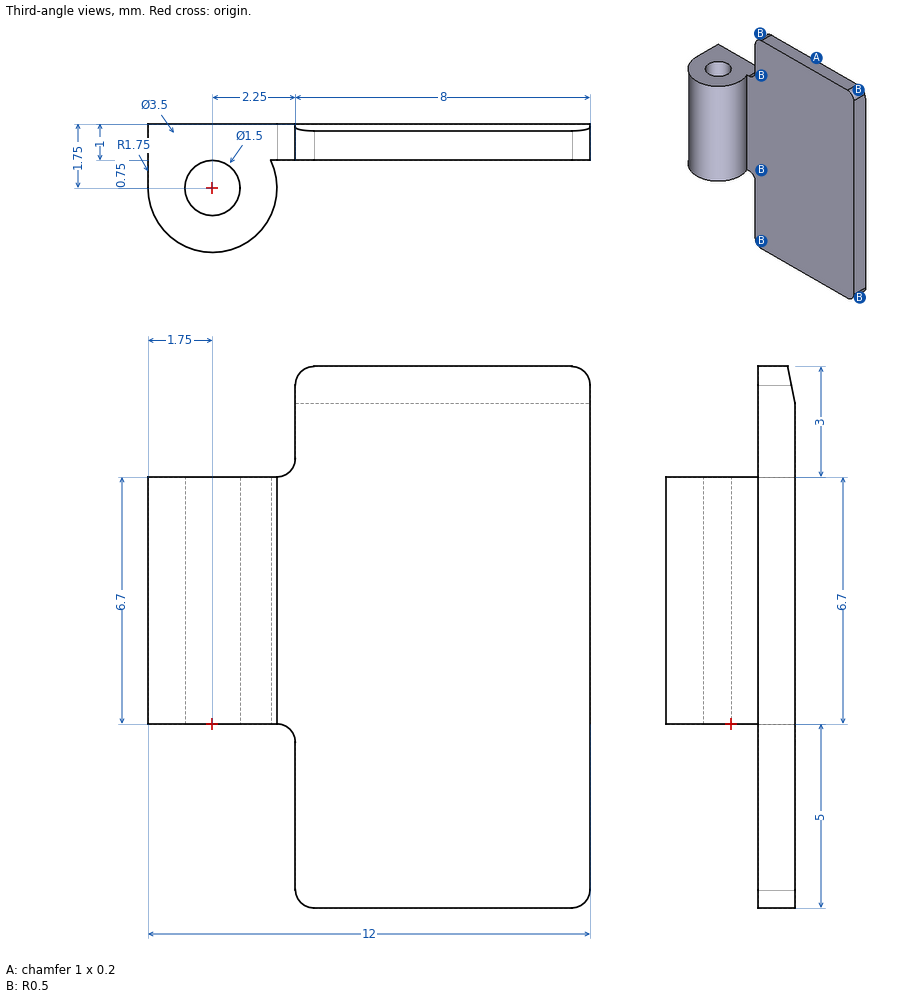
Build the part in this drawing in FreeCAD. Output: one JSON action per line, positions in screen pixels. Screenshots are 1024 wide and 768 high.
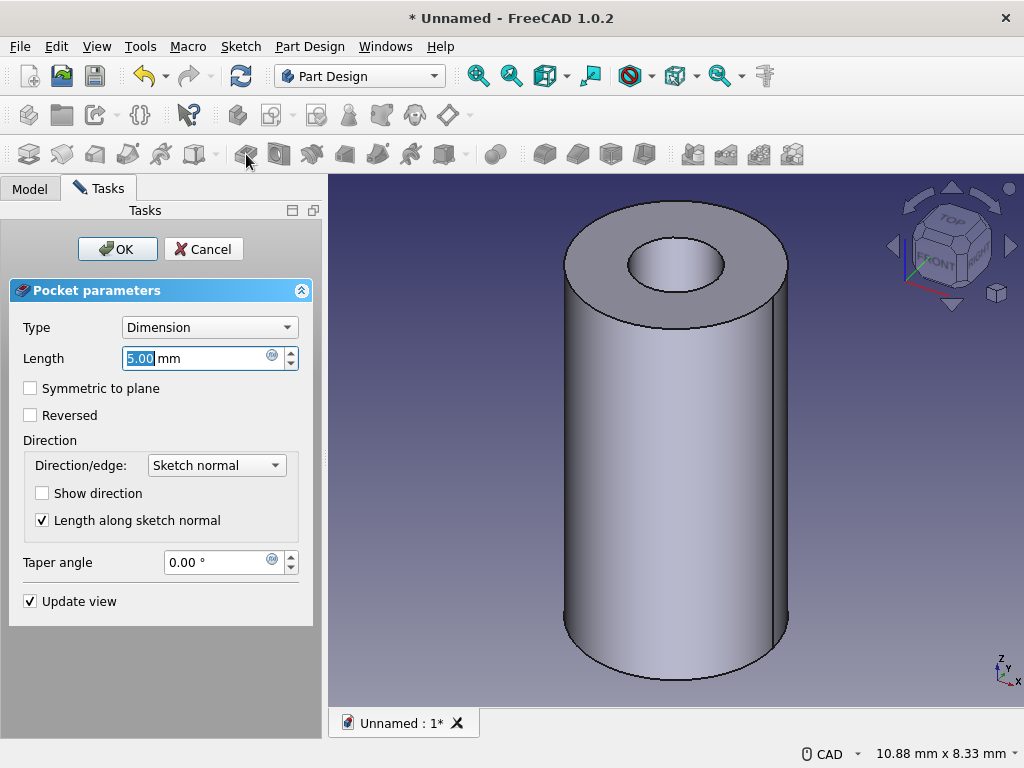
{"action": "left_click", "coordinate": [210, 328]}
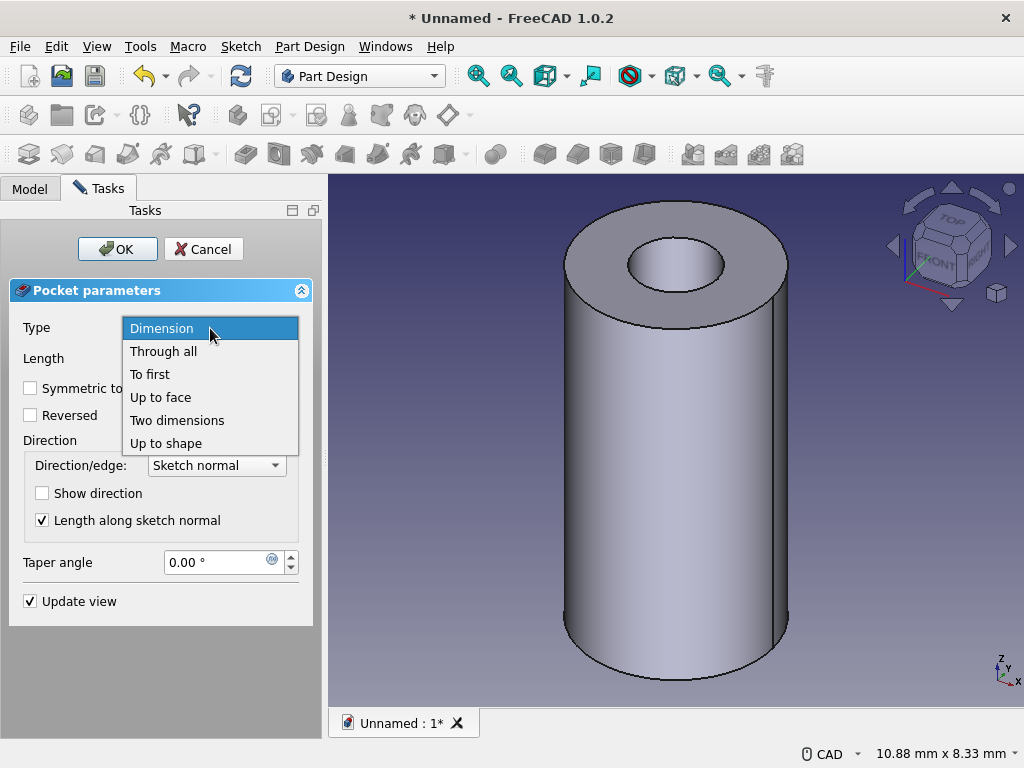
{"action": "left_click", "coordinate": [208, 352]}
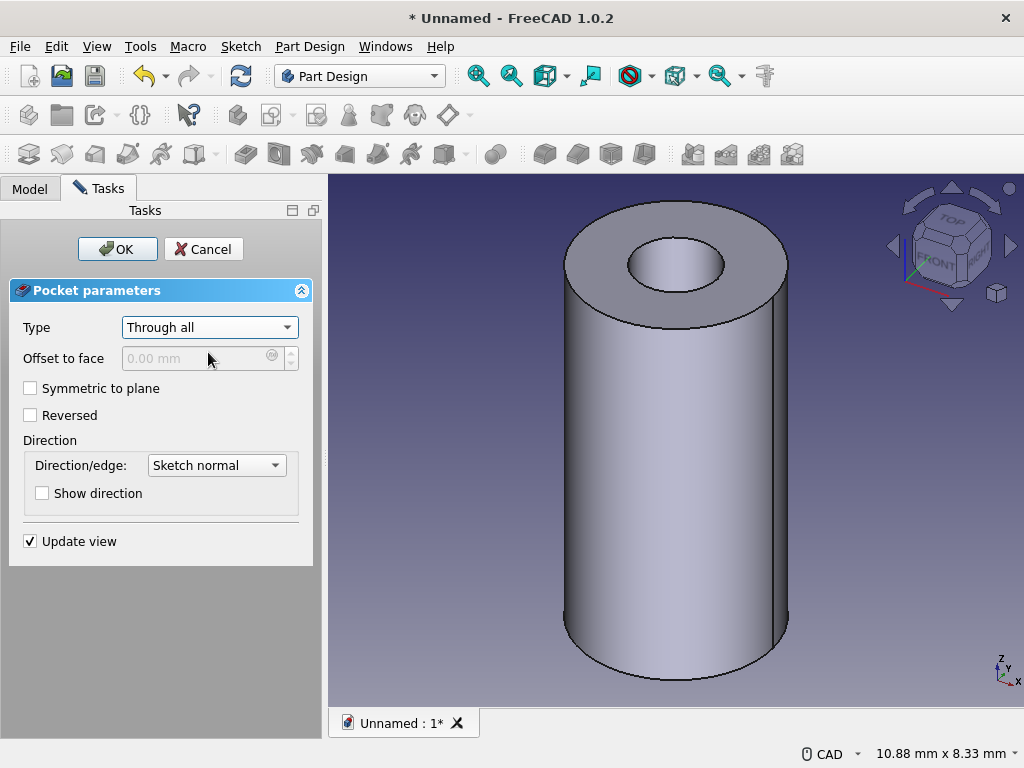
{"action": "left_click", "coordinate": [118, 249]}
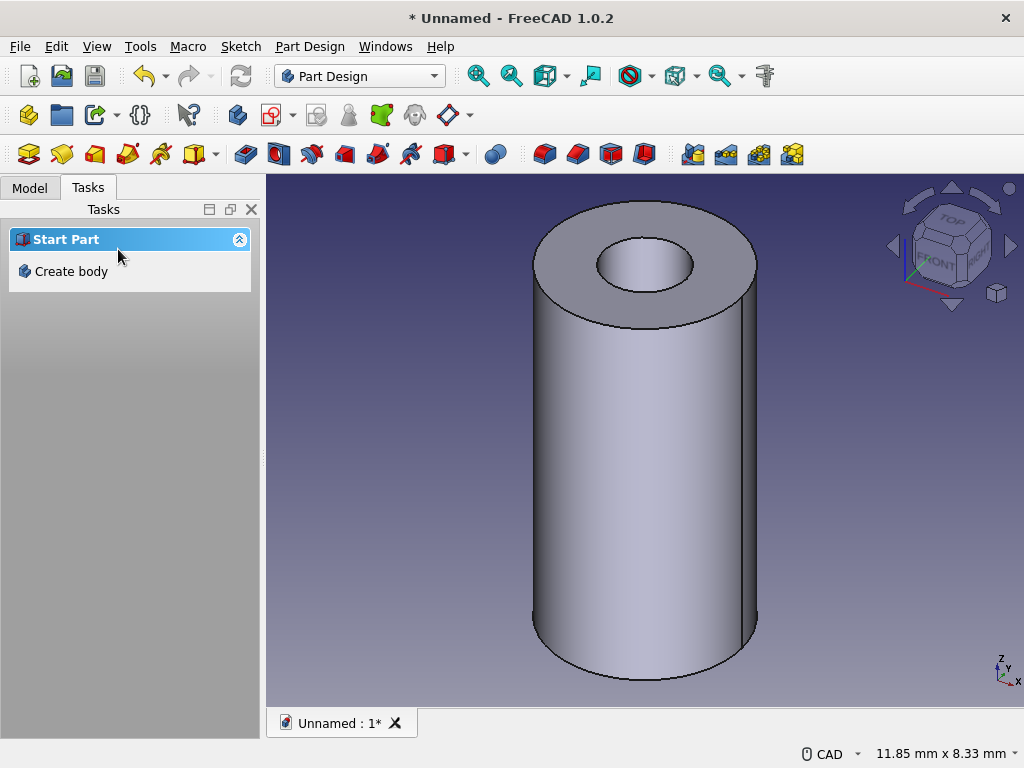
{"action": "left_click", "coordinate": [30, 188]}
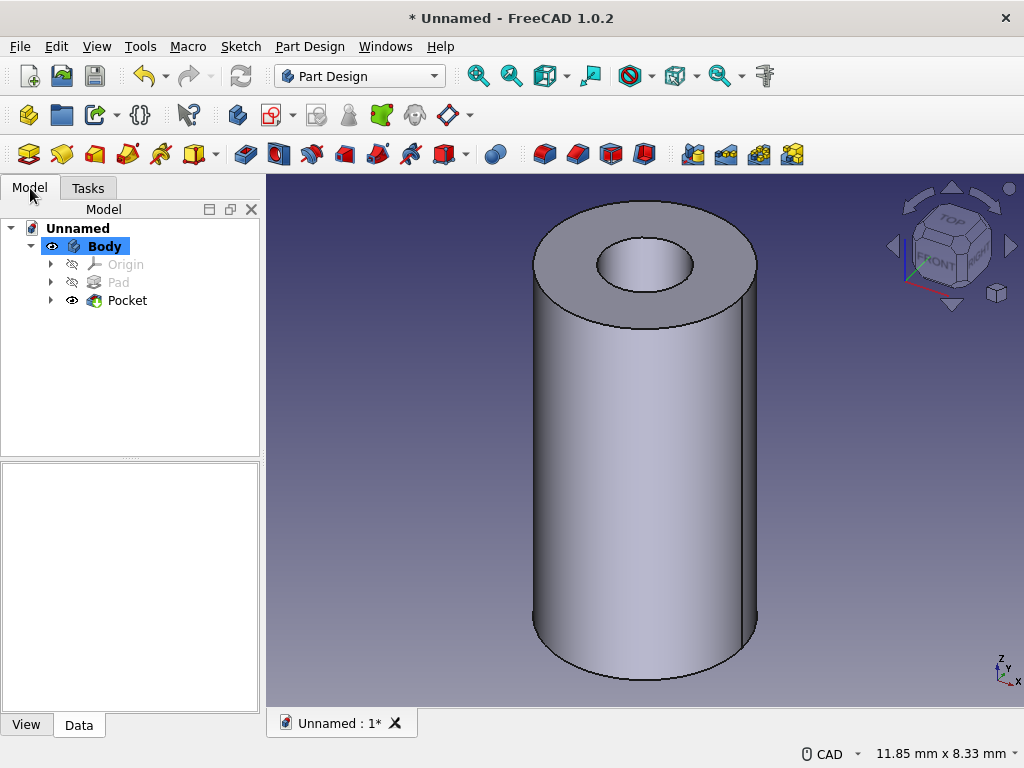
{"action": "left_click", "coordinate": [51, 264]}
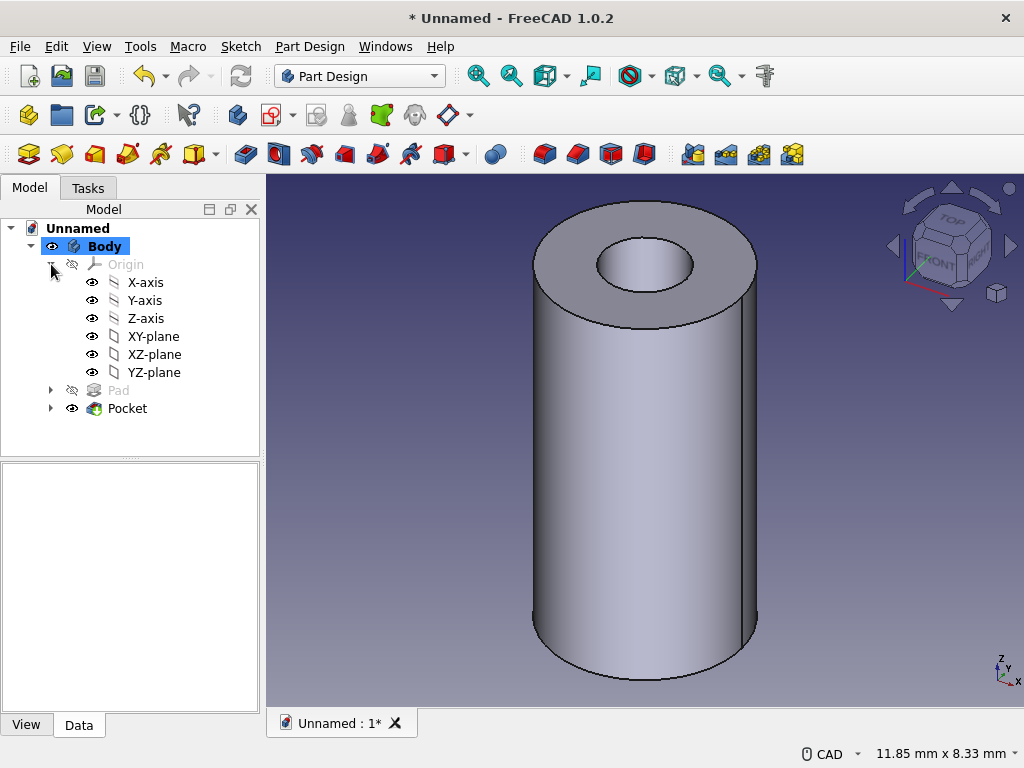
{"action": "left_click", "coordinate": [137, 354]}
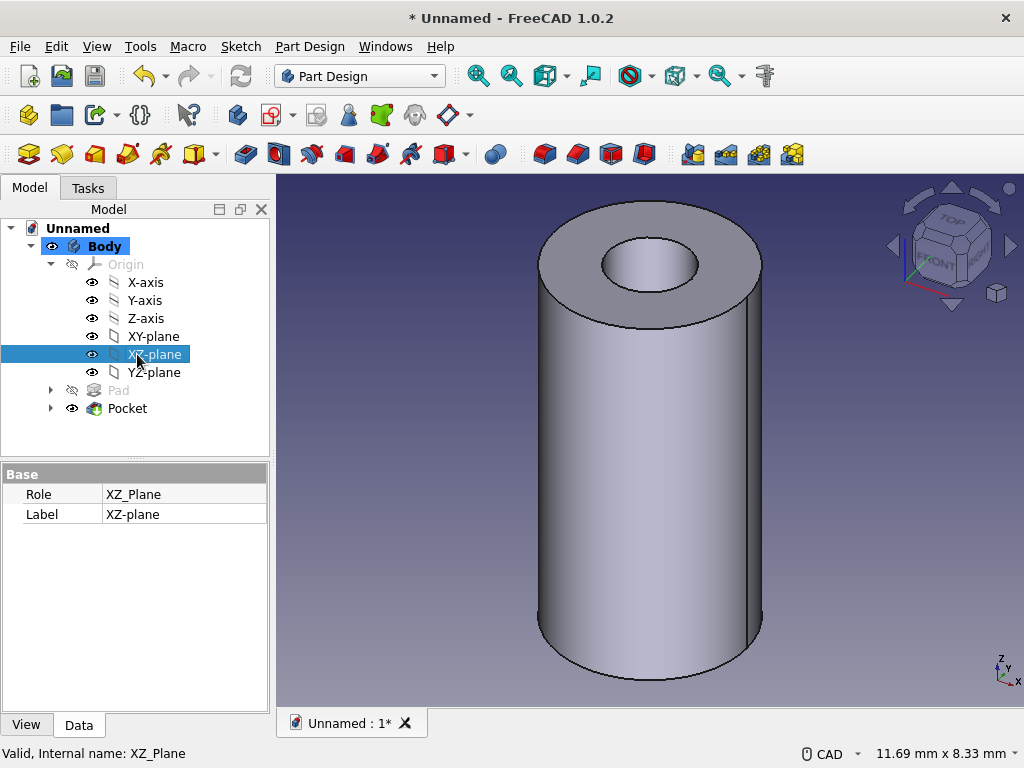
{"action": "left_click", "coordinate": [448, 116]}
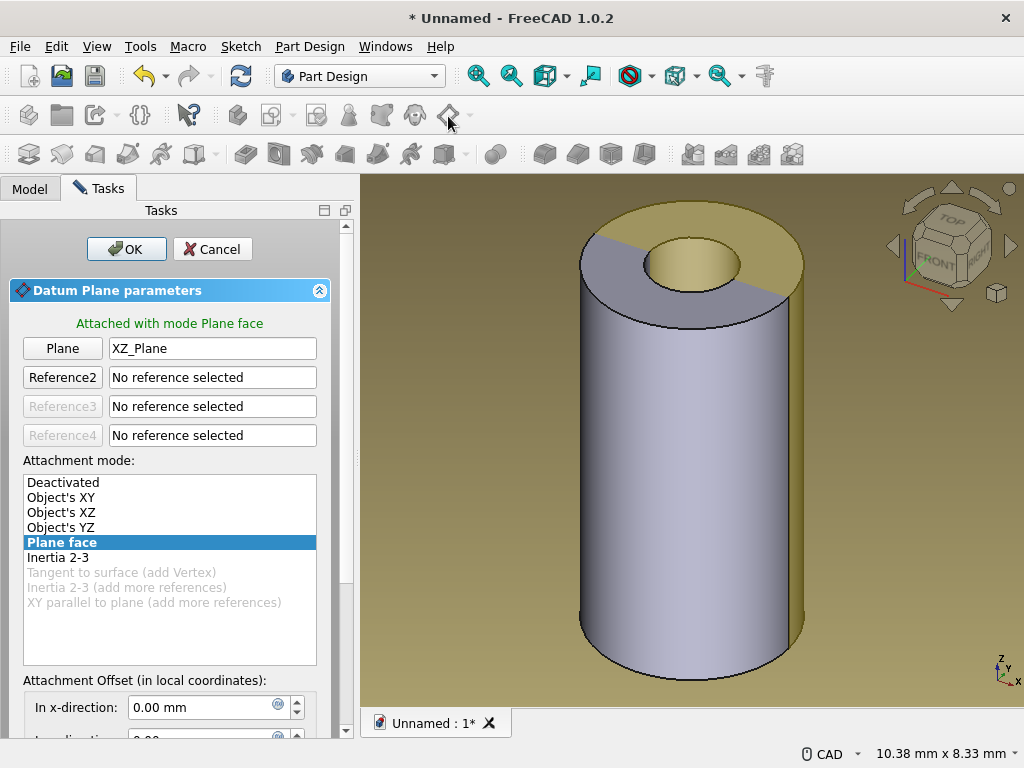
{"action": "scroll", "coordinate": [346, 479], "scroll_direction": "down", "scroll_amount": 2}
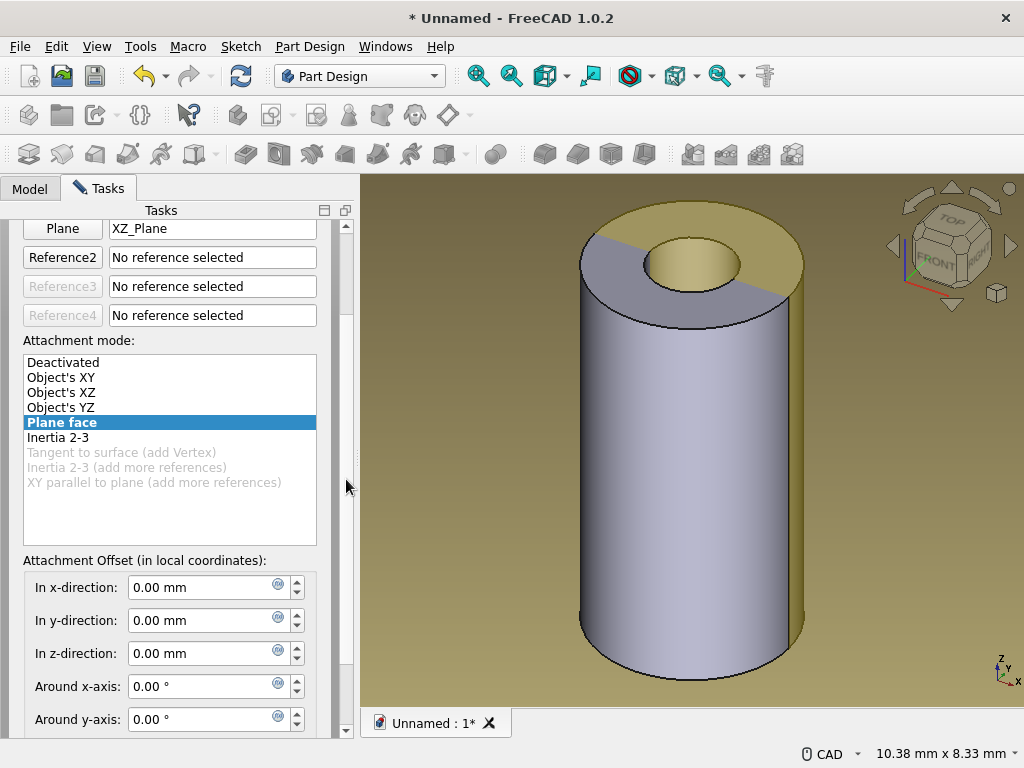
{"action": "triple_click", "coordinate": [210, 654]}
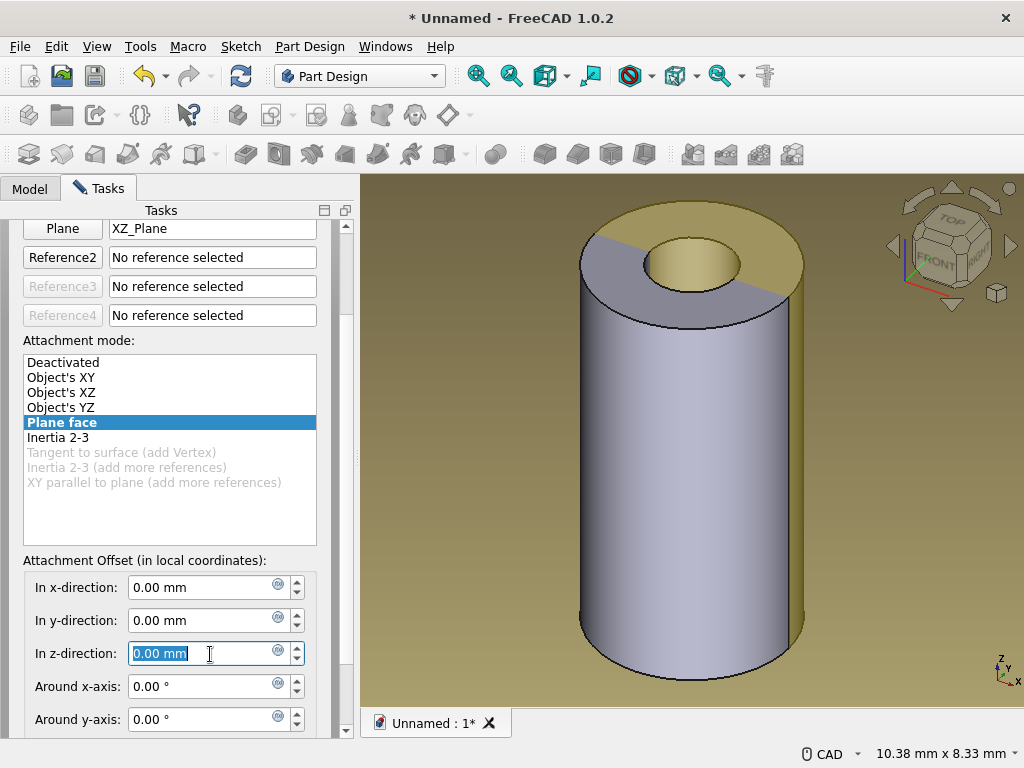
{"action": "type", "text": "-1.75"}
{"action": "key", "text": "Tab"}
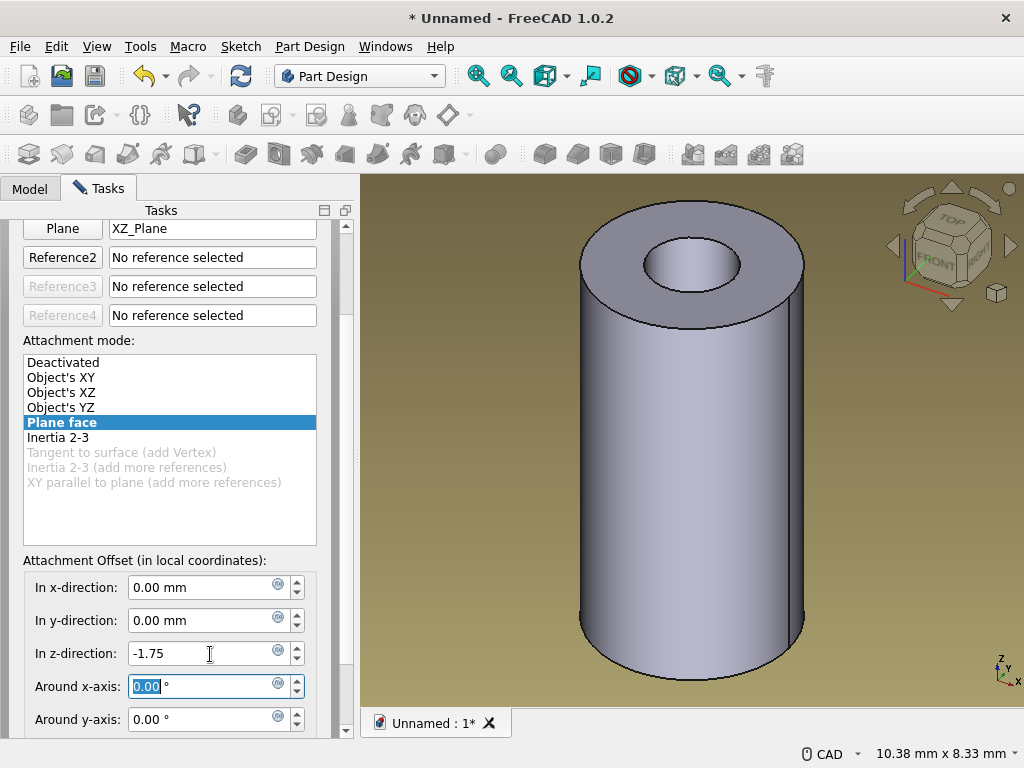
{"action": "scroll", "coordinate": [346, 479], "scroll_direction": "up", "scroll_amount": 3}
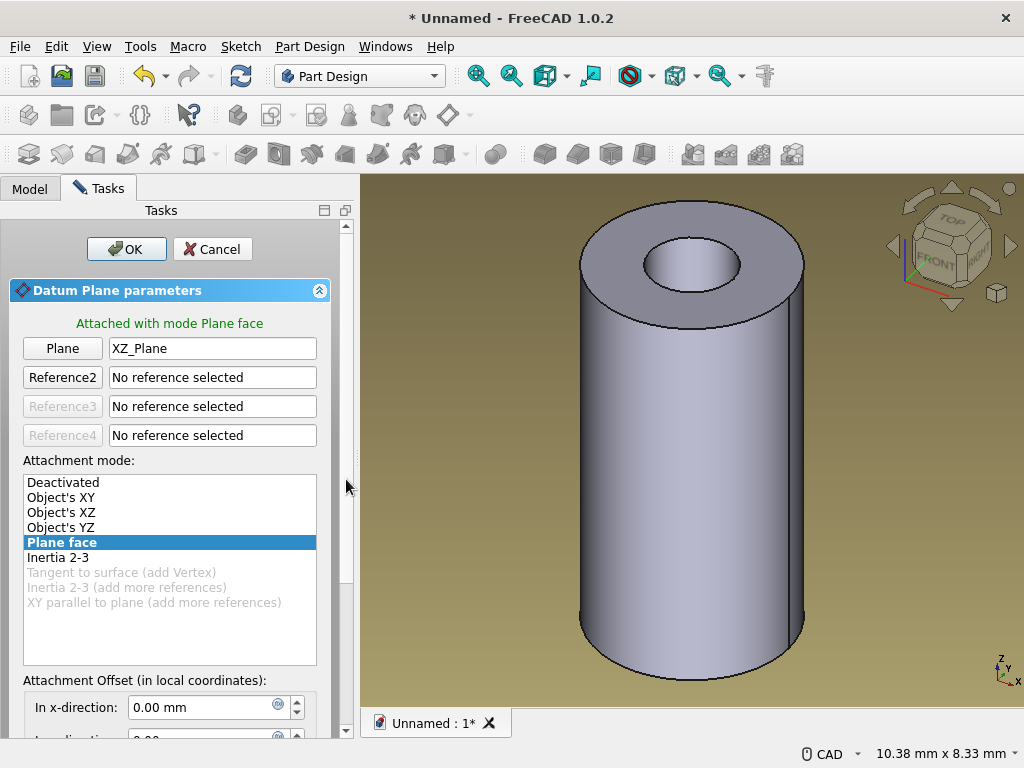
{"action": "left_click", "coordinate": [127, 249]}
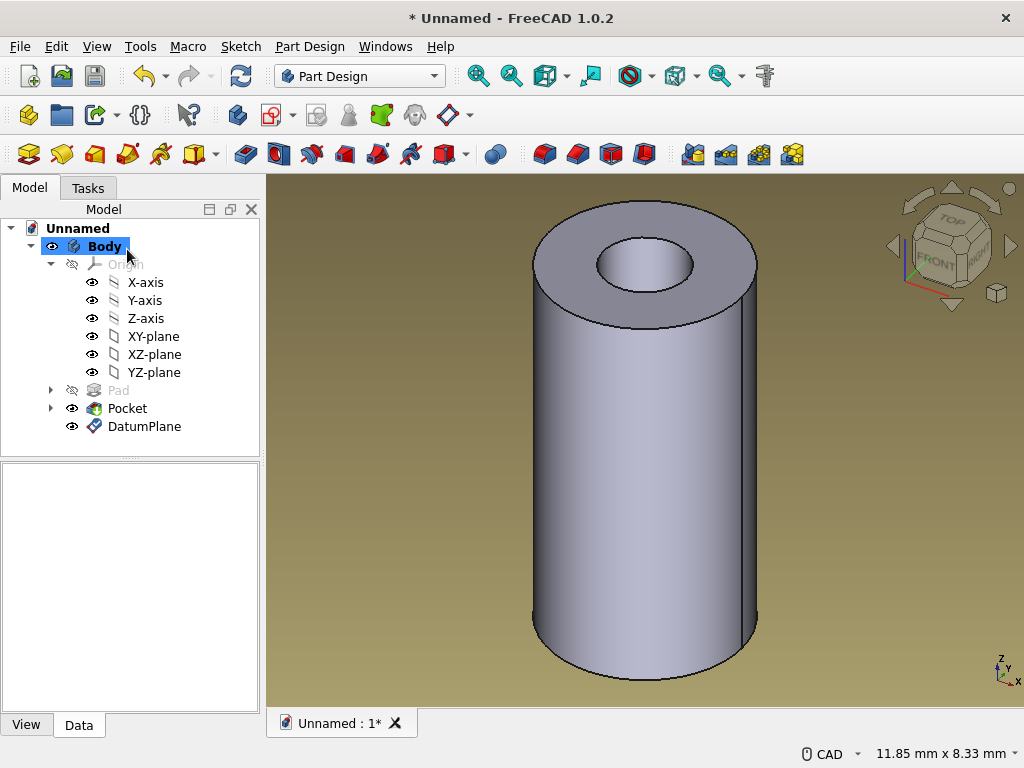
{"action": "left_click", "coordinate": [117, 426]}